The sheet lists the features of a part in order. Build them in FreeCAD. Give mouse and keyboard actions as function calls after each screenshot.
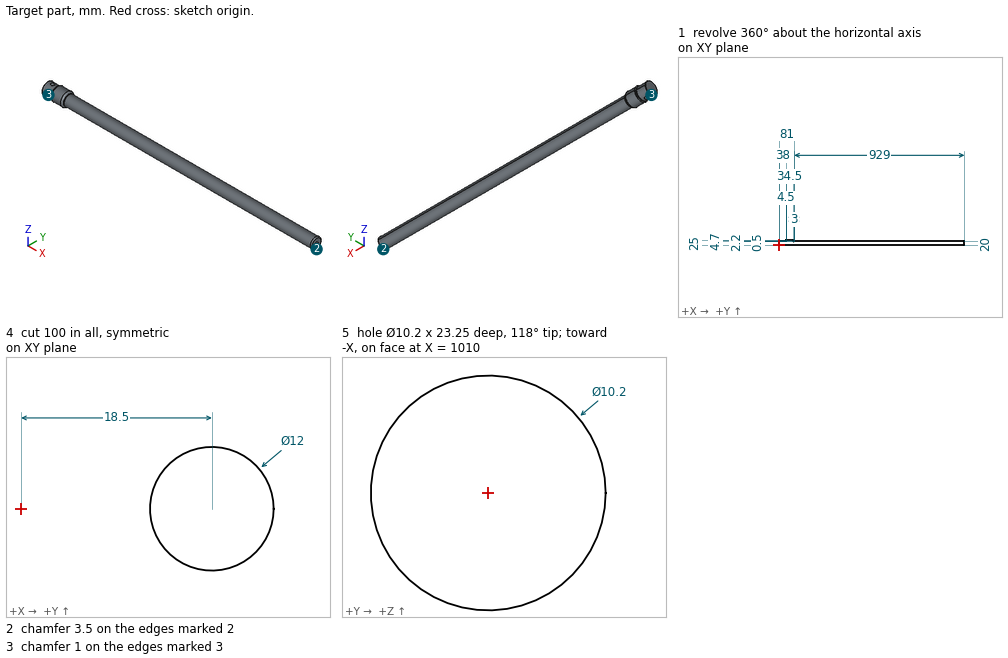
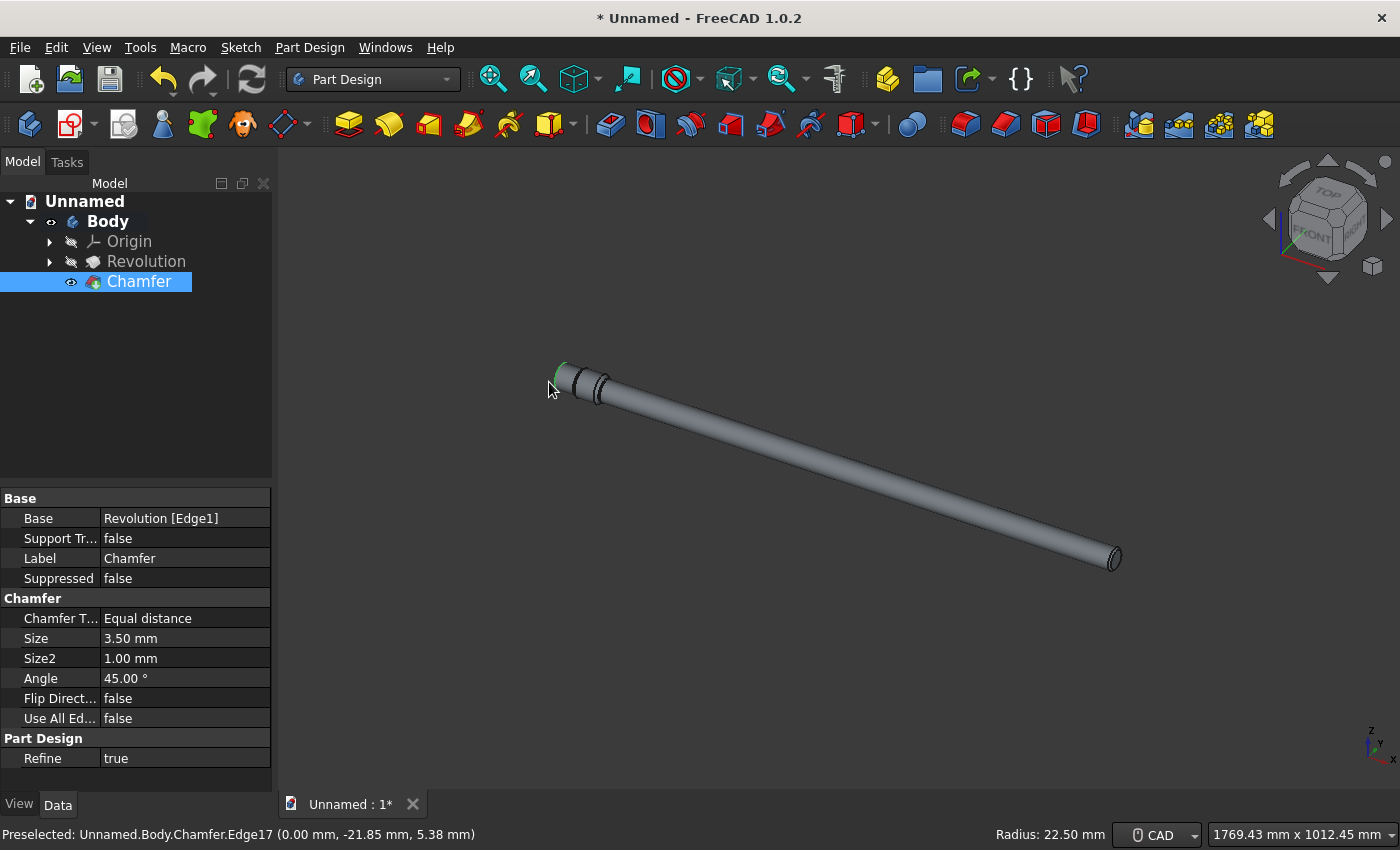
click(1006, 124)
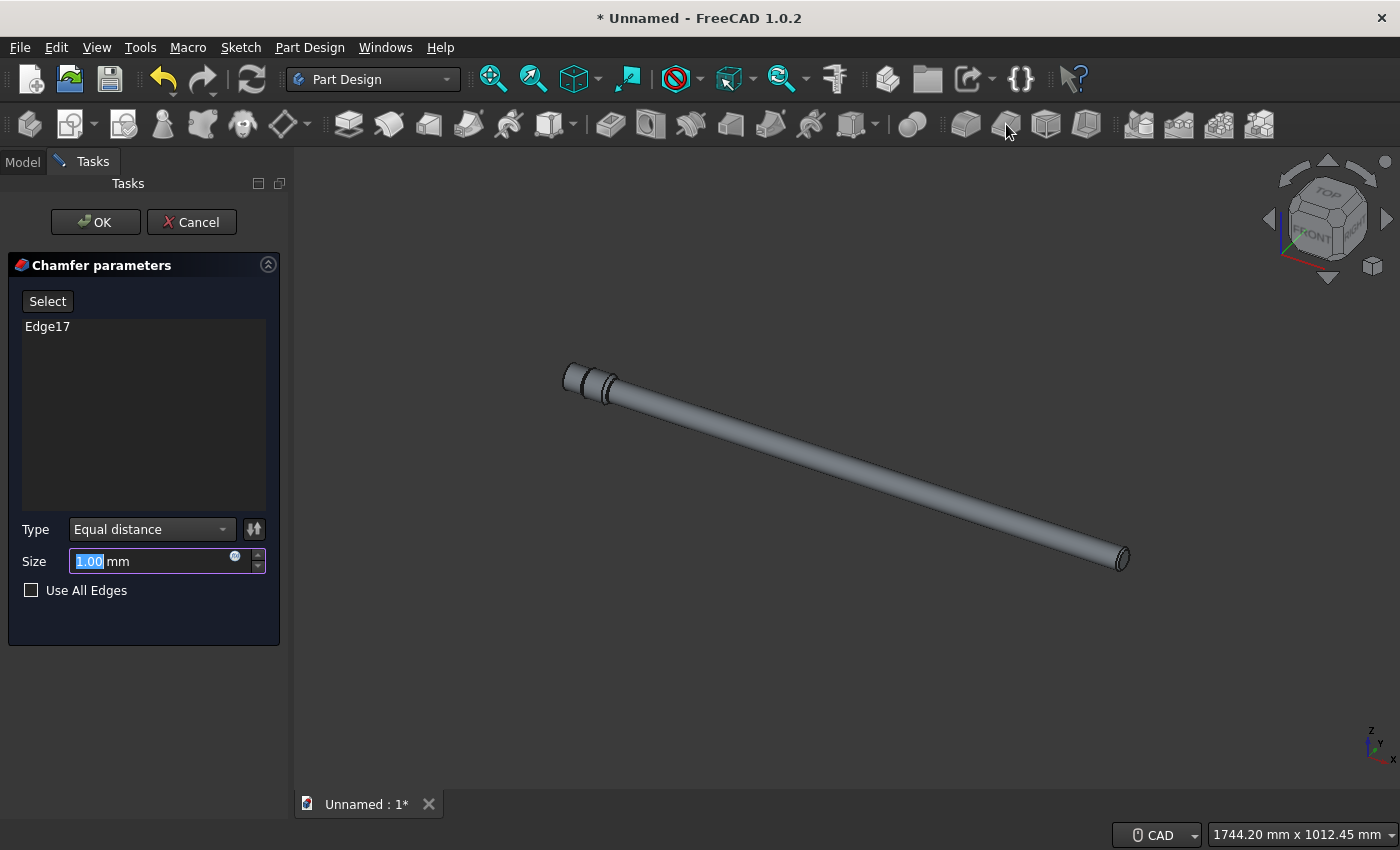
text(1)
key(Tab)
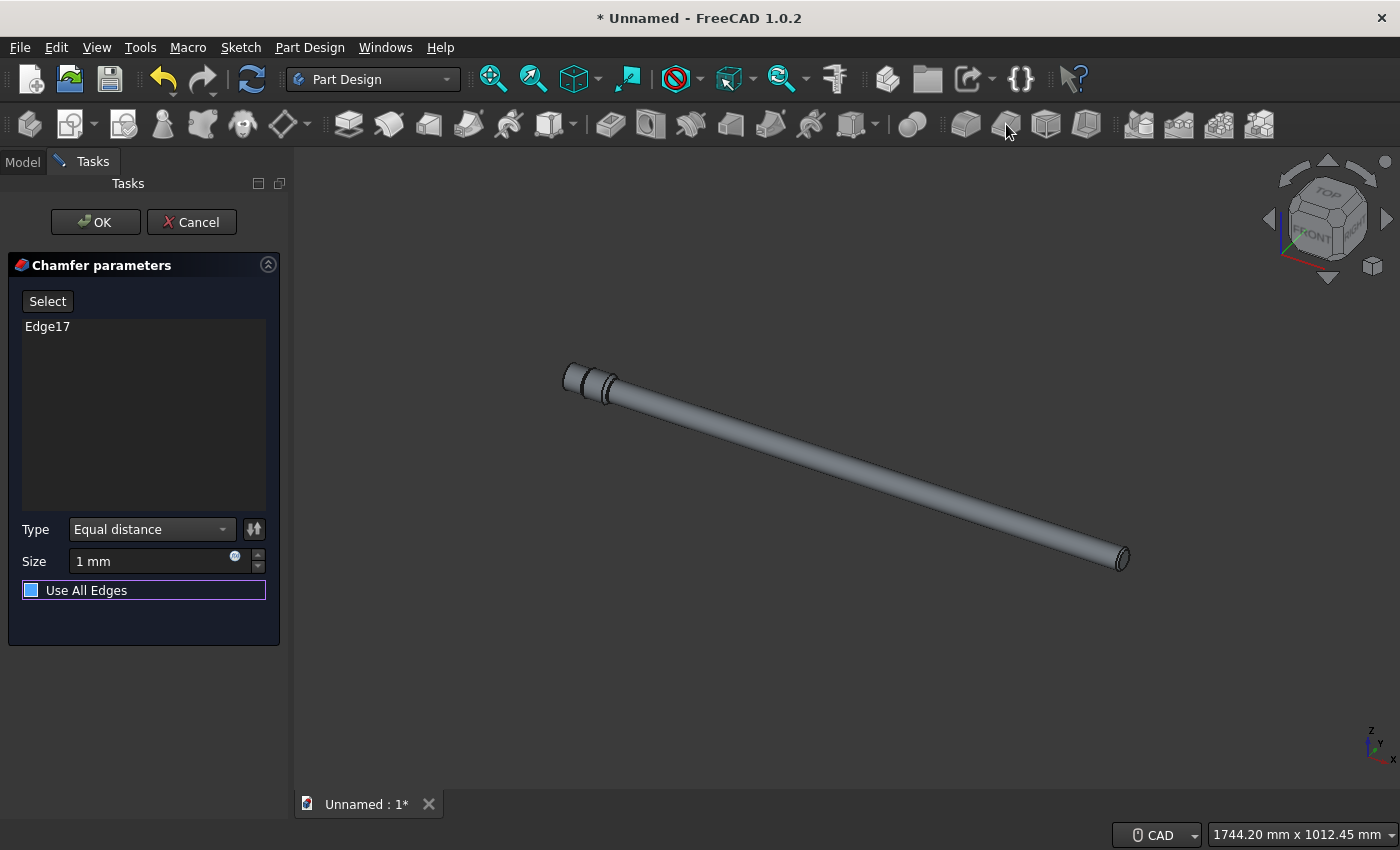
click(96, 222)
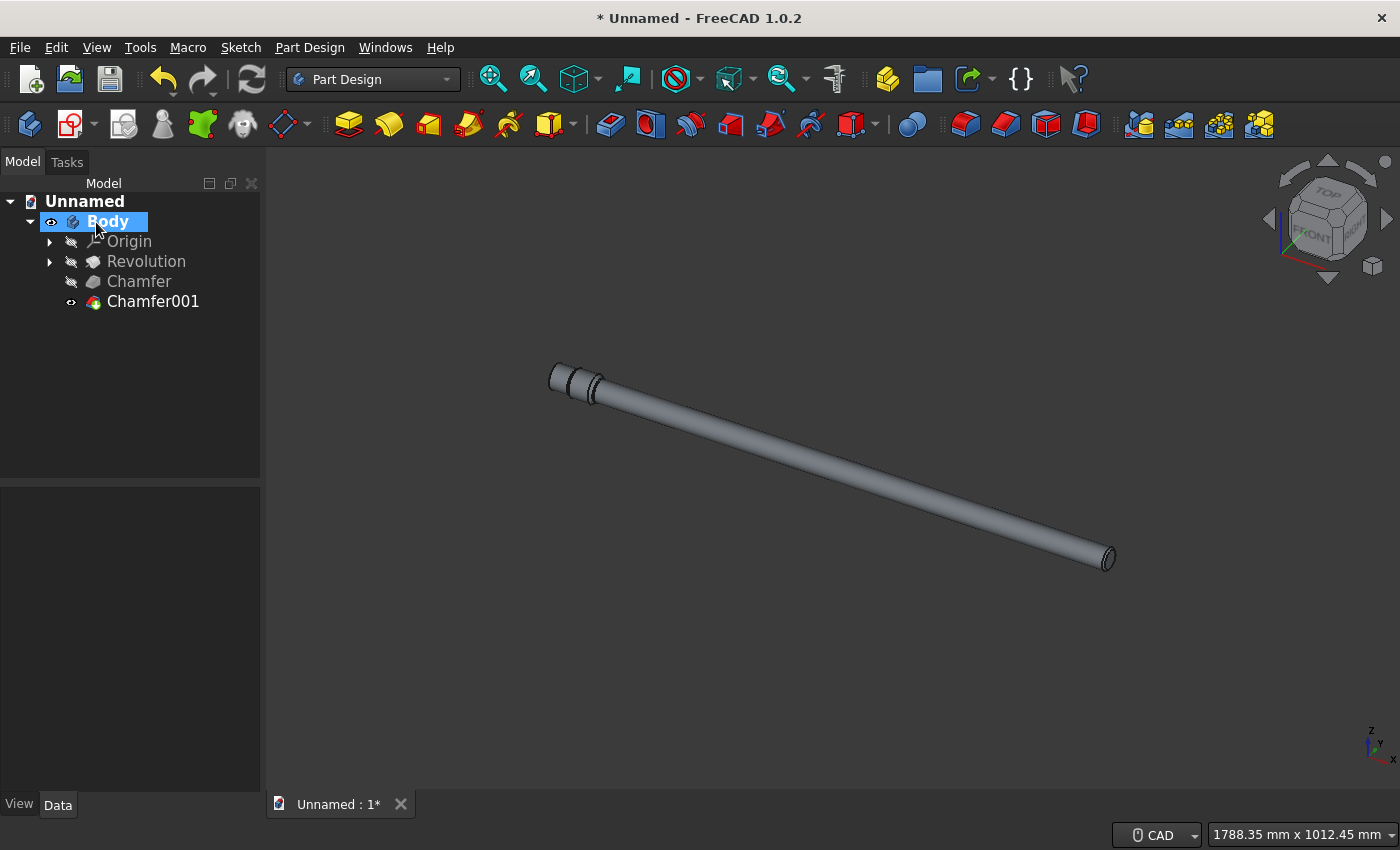
click(70, 124)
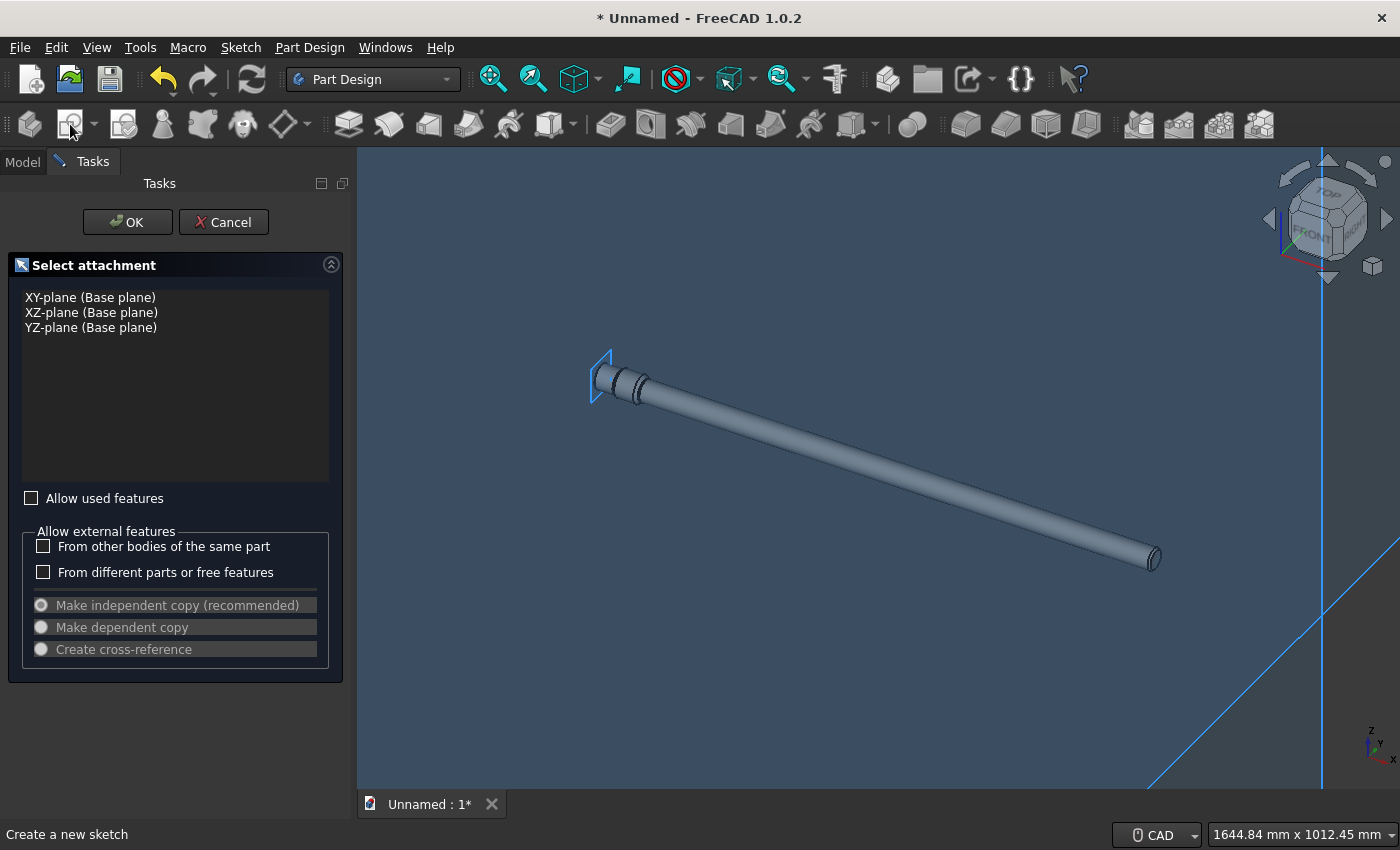
click(82, 298)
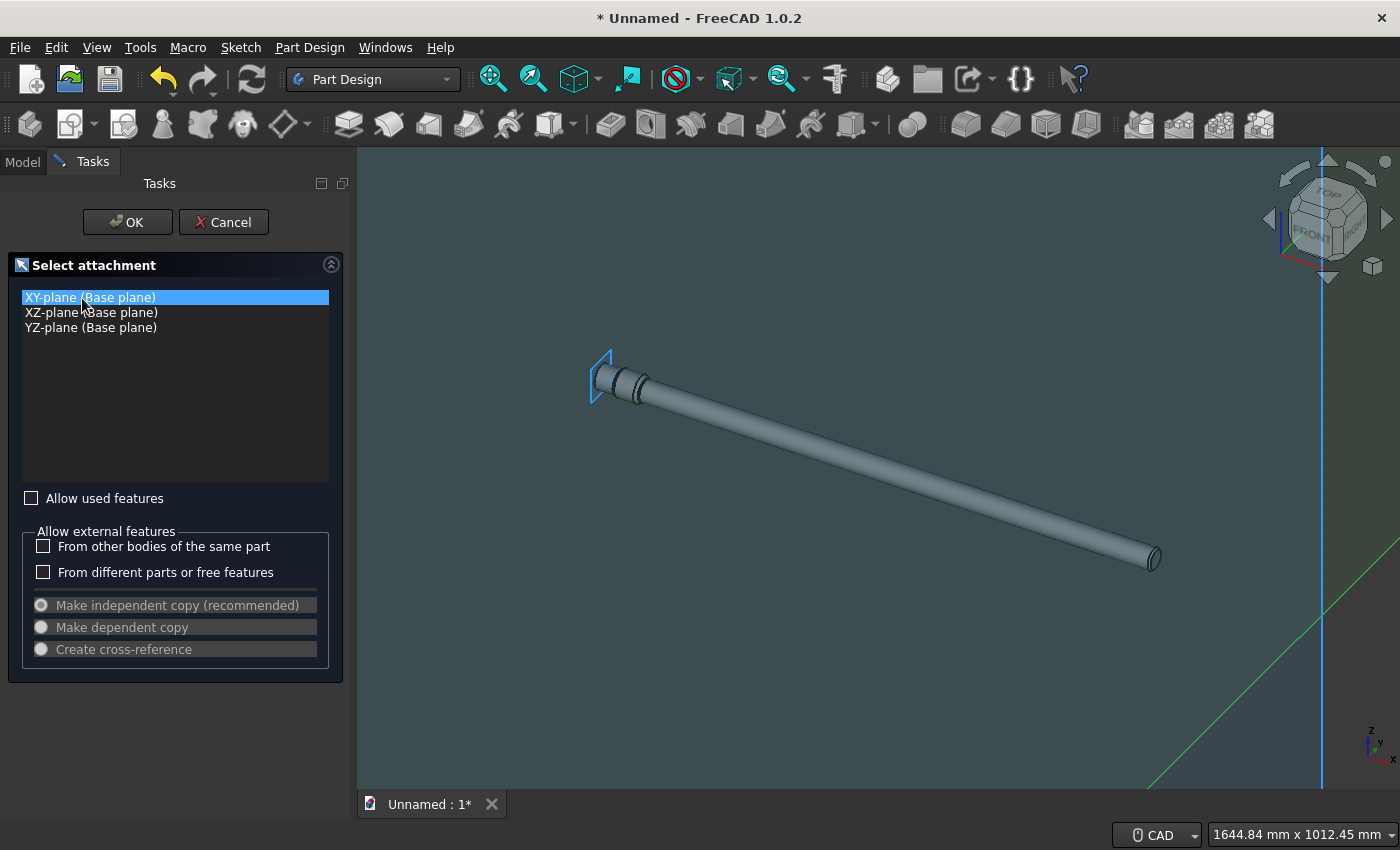
click(128, 222)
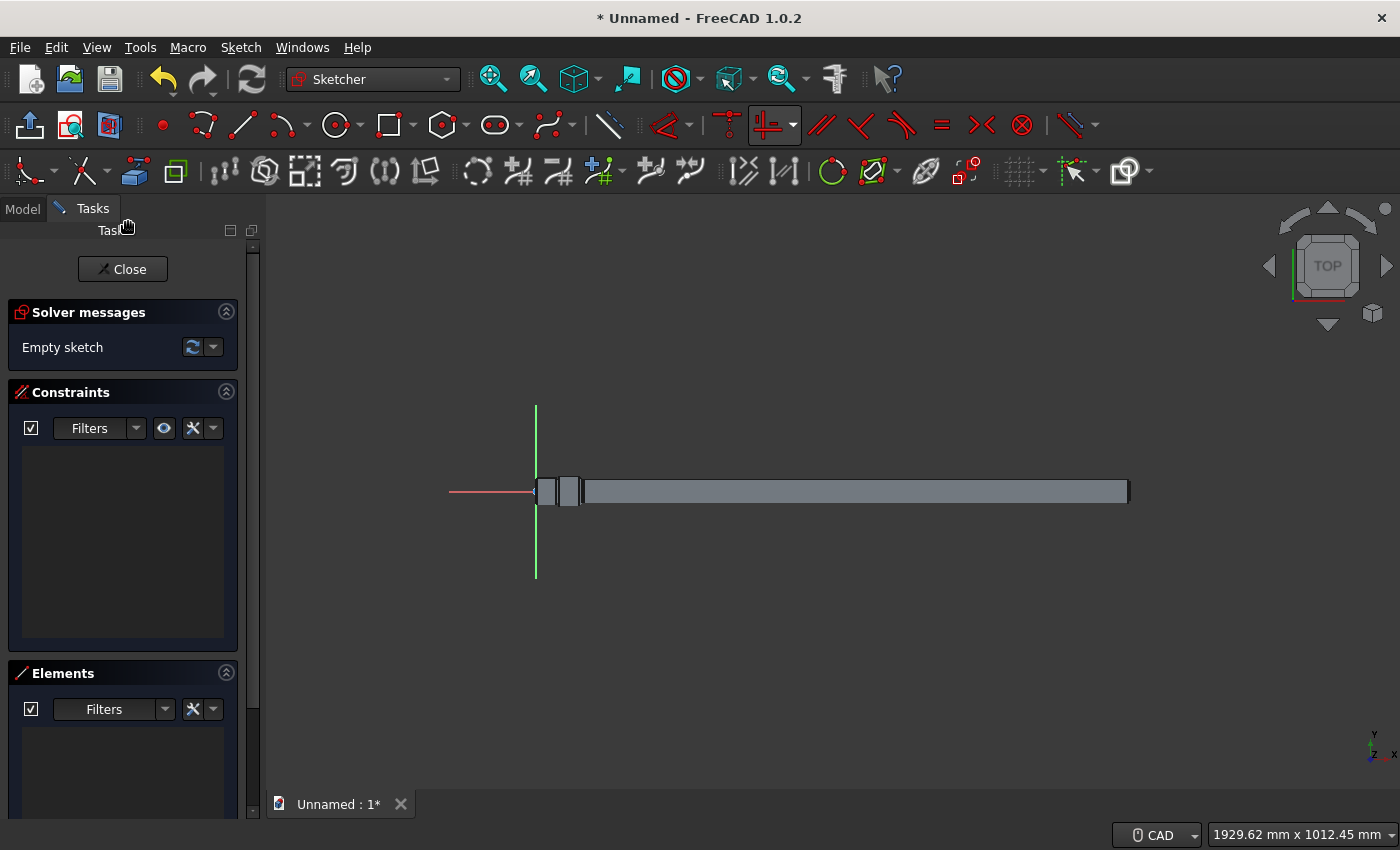
click(110, 126)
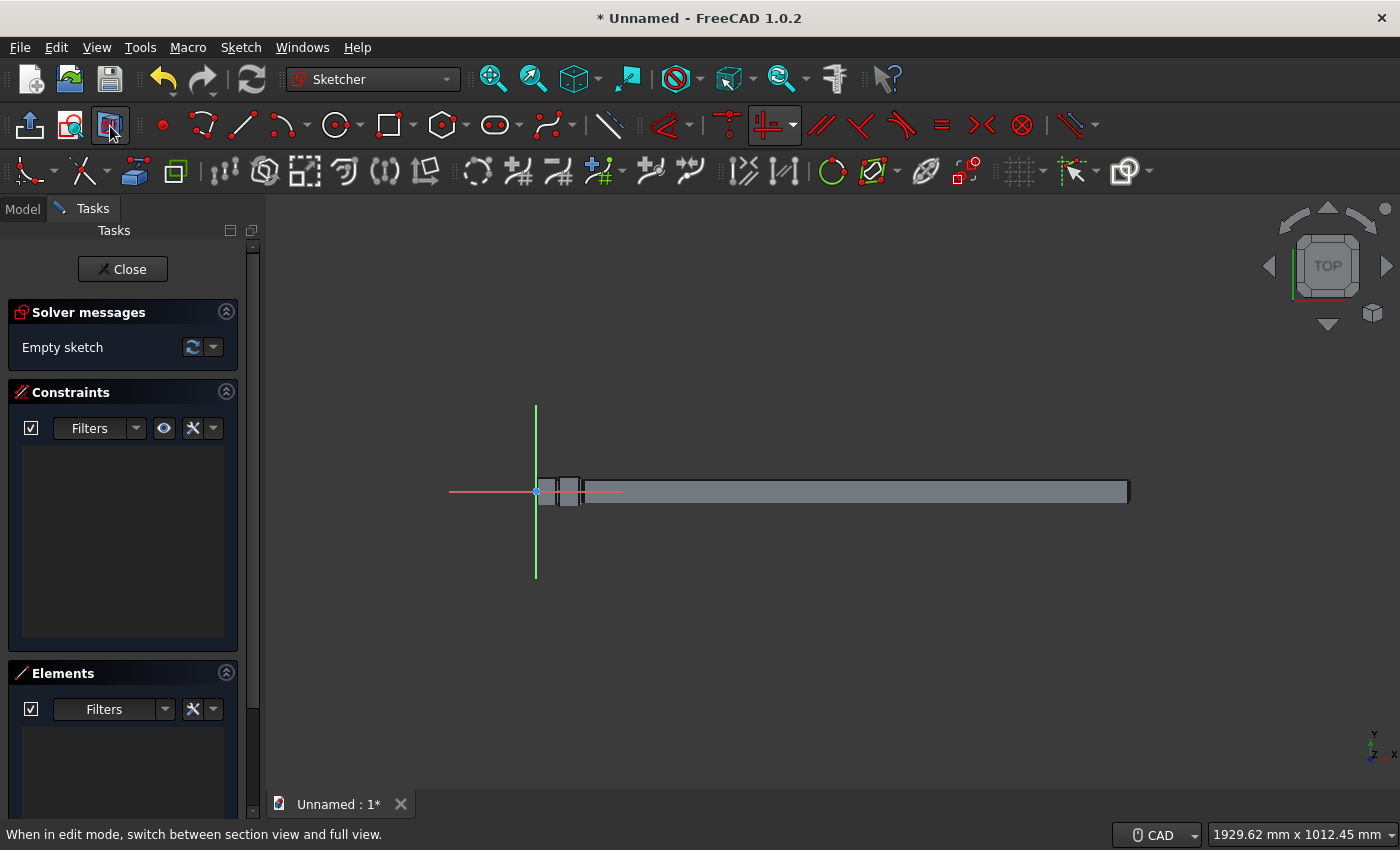
scroll(532, 492, up, 15)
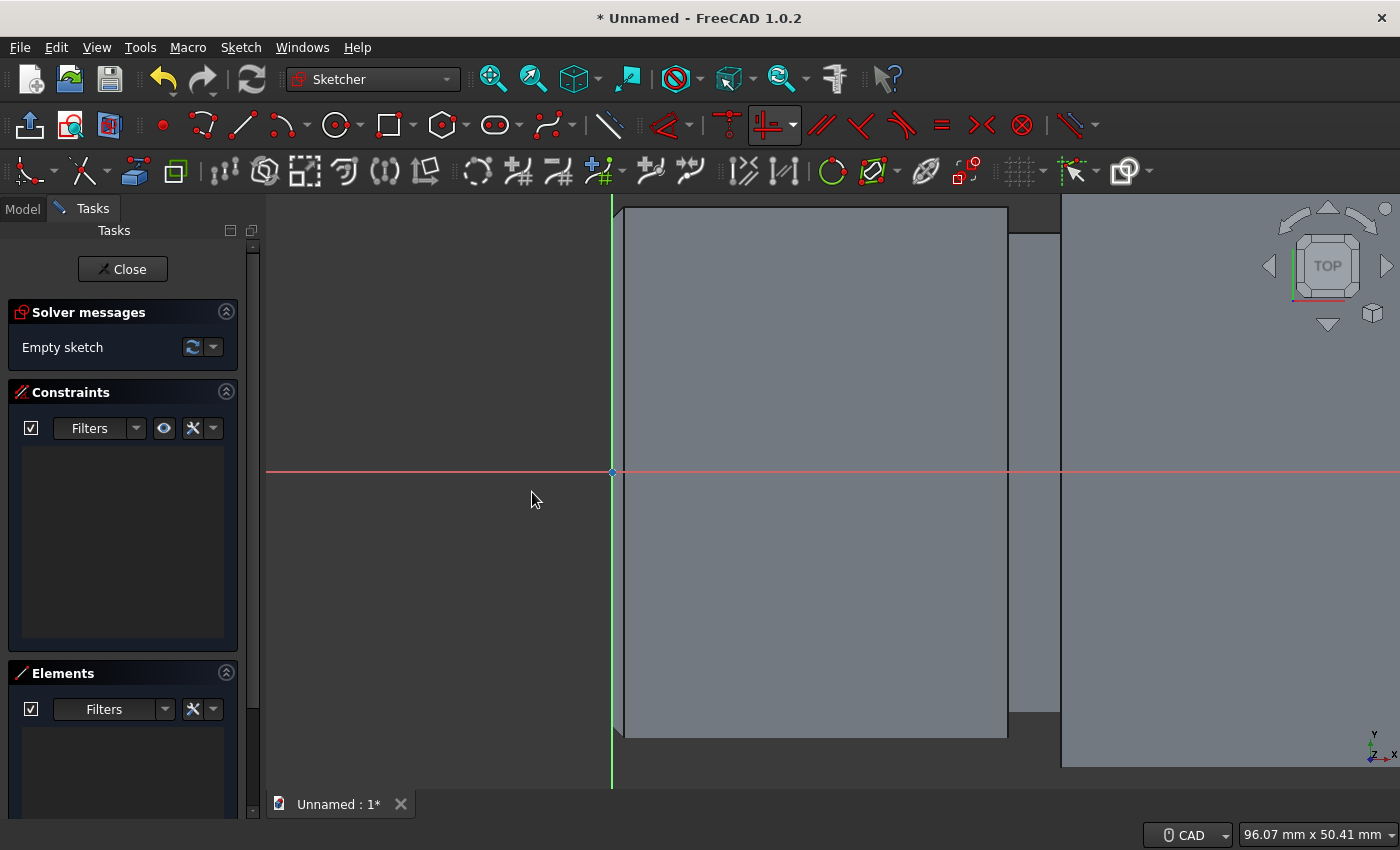
scroll(751, 457, up, 4)